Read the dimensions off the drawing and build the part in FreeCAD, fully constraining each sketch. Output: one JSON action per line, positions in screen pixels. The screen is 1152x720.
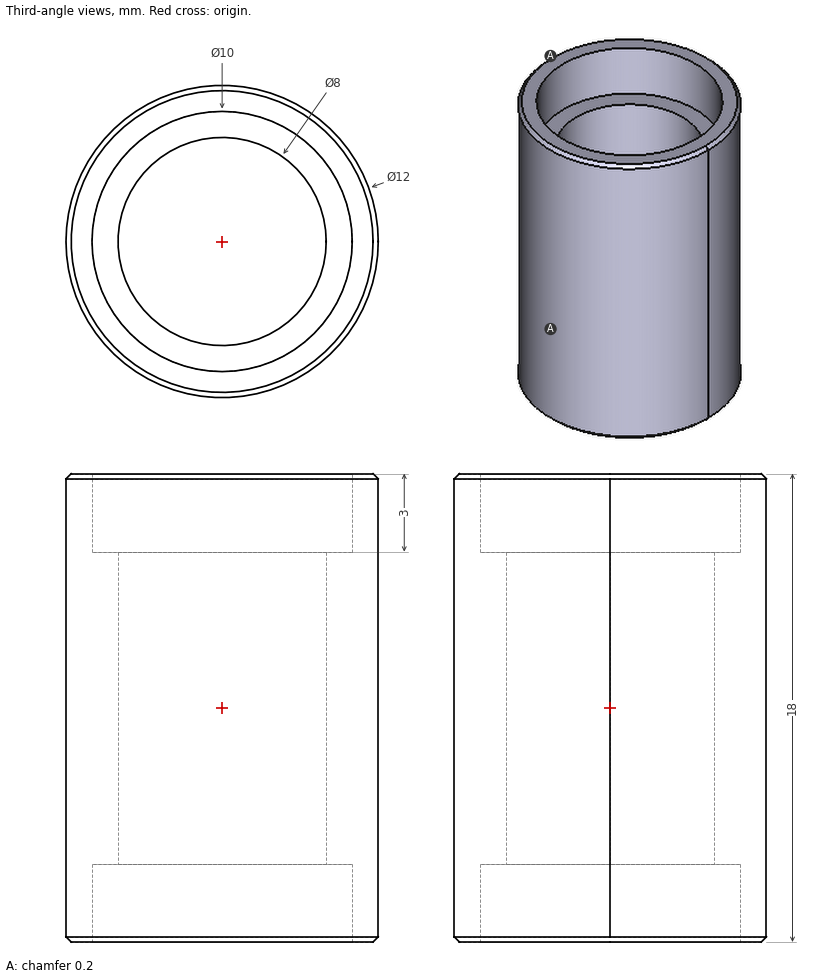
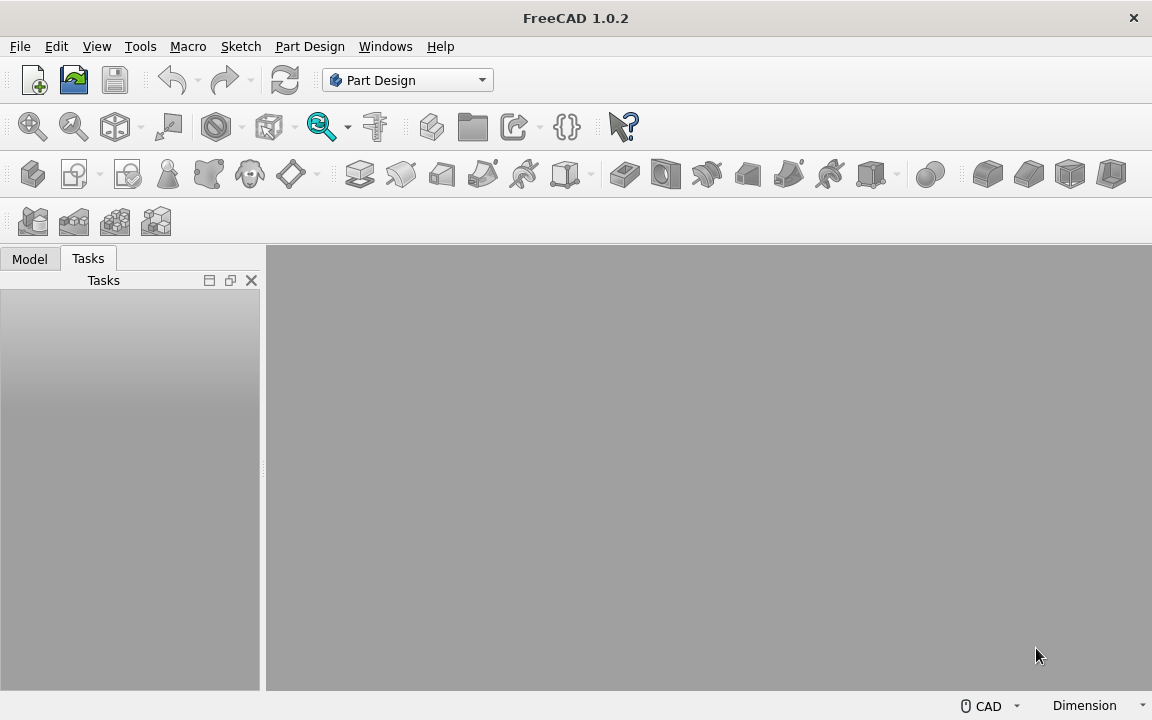
{"action": "left_click", "coordinate": [33, 80]}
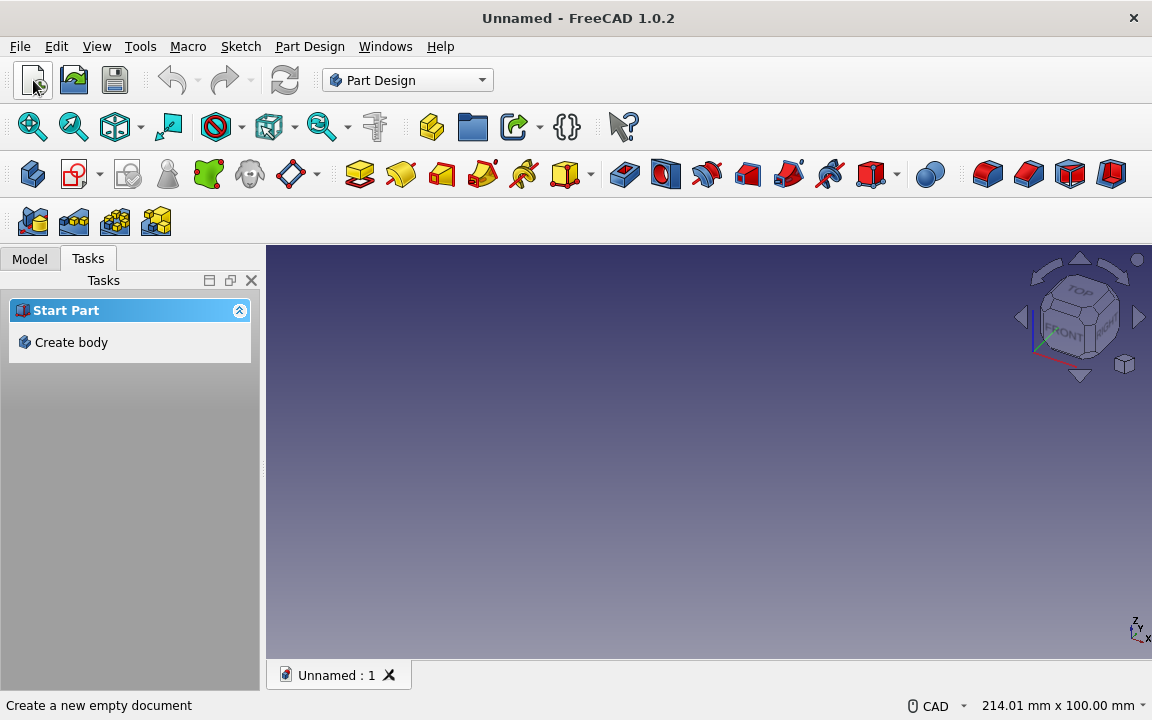
{"action": "left_click", "coordinate": [74, 174]}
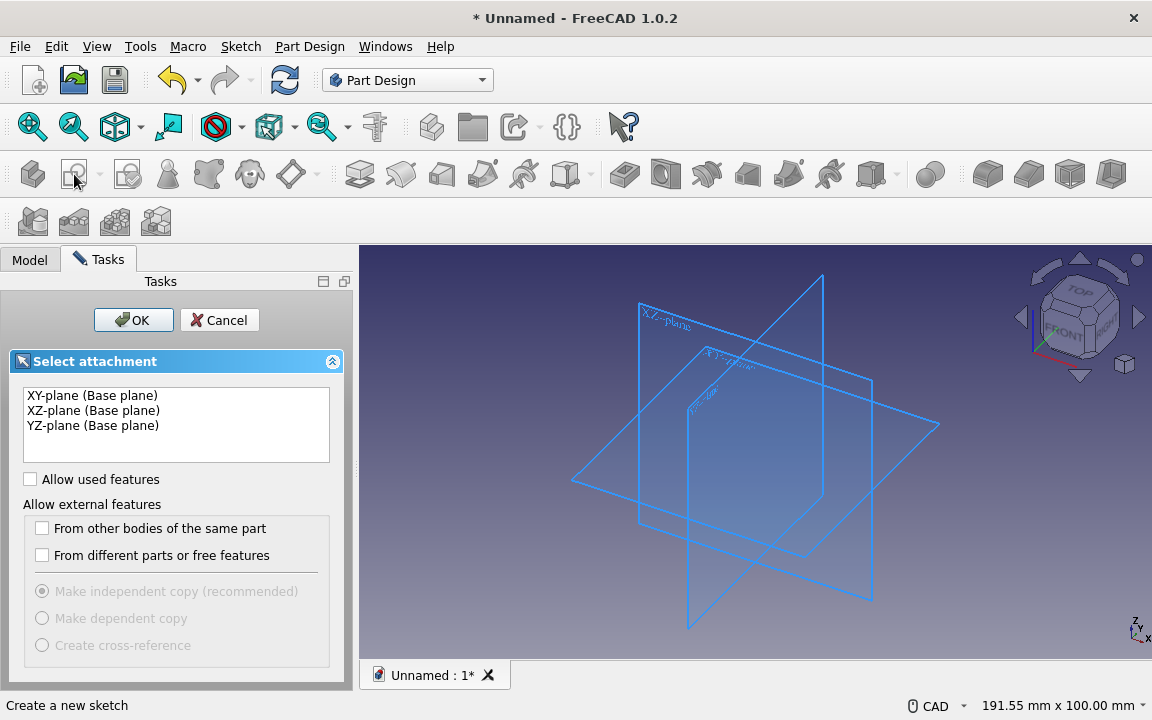
{"action": "left_click", "coordinate": [84, 396]}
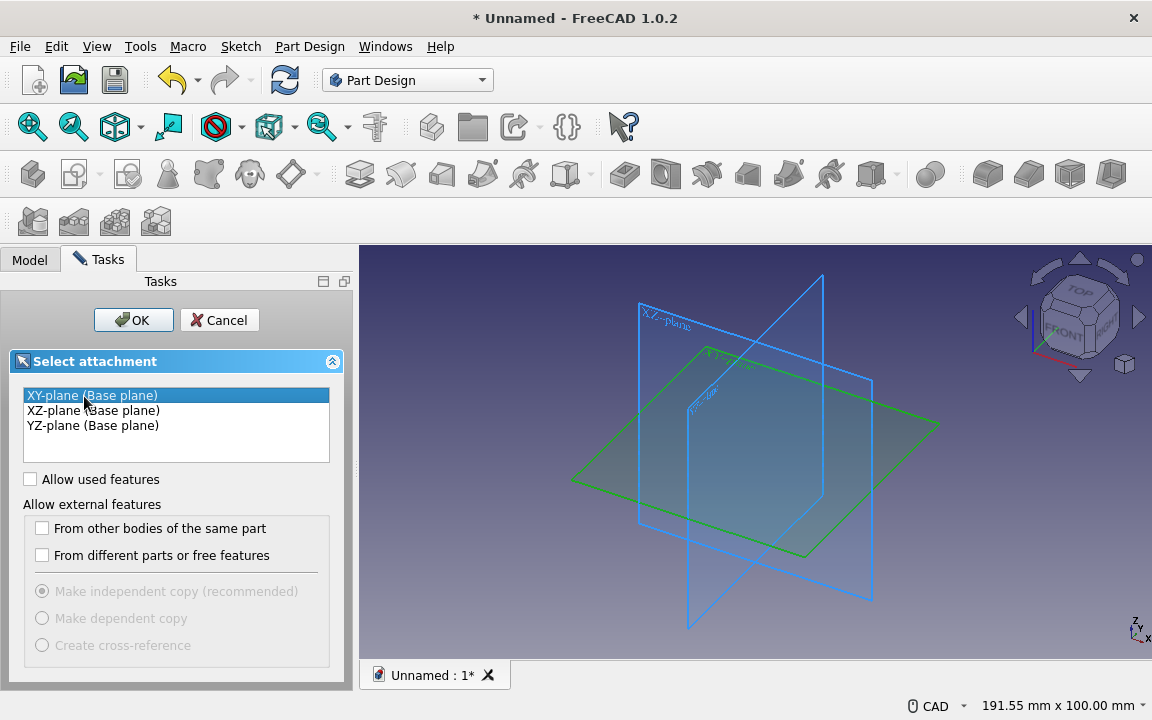
{"action": "left_click", "coordinate": [134, 320]}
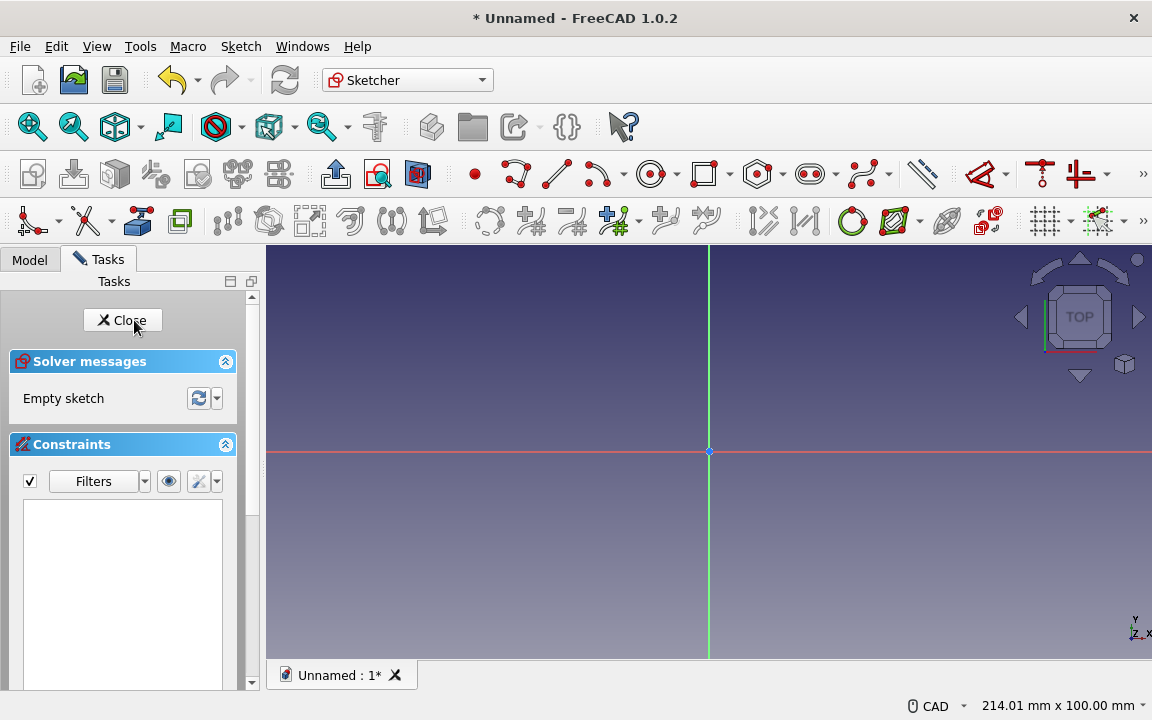
{"action": "scroll", "coordinate": [726, 452], "scroll_direction": "up", "scroll_amount": 8}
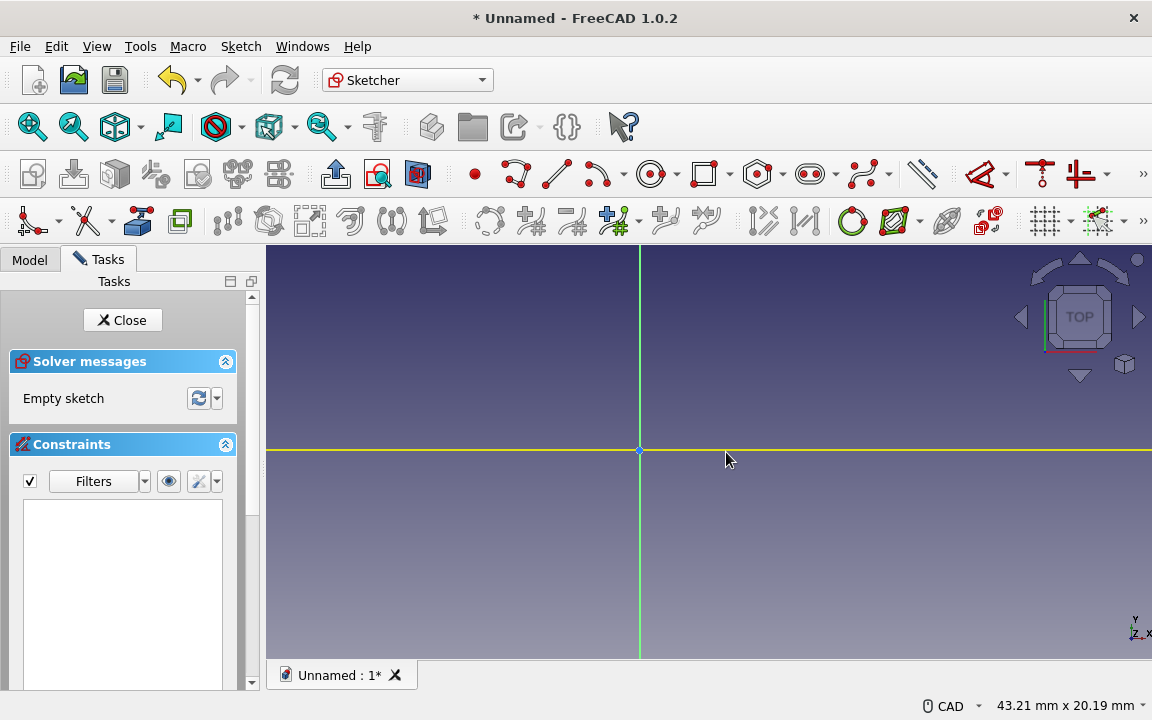
{"action": "left_click", "coordinate": [650, 174]}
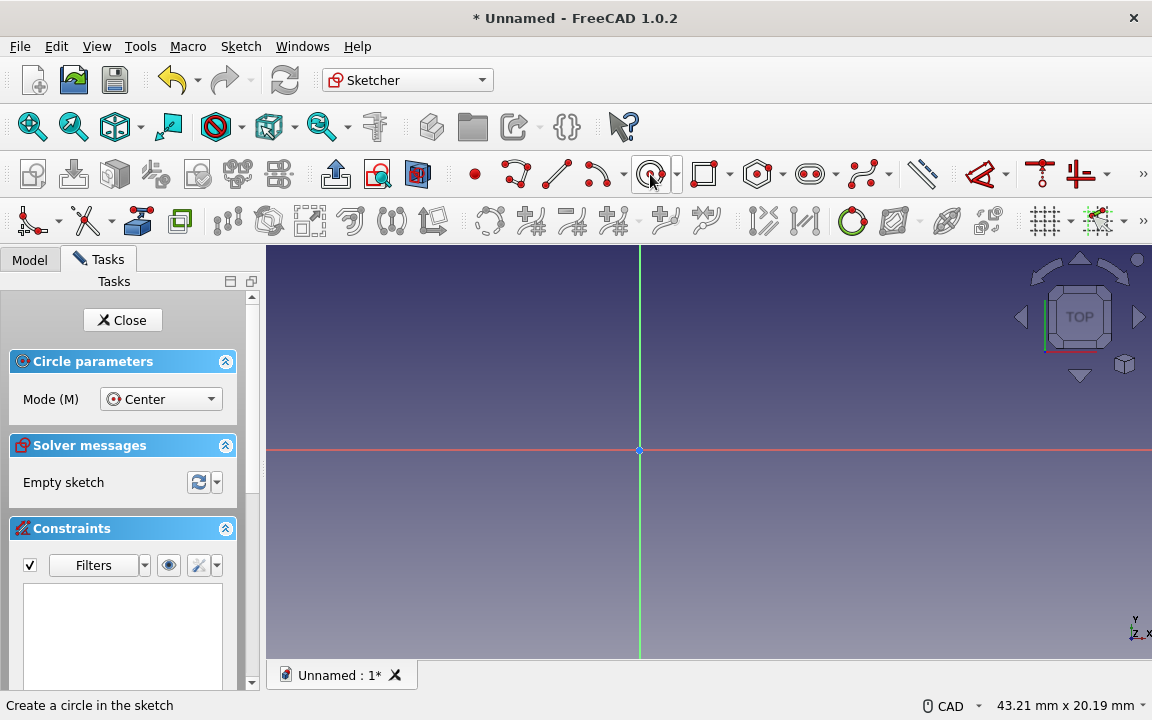
{"action": "left_click", "coordinate": [640, 450]}
{"action": "left_click", "coordinate": [727, 363]}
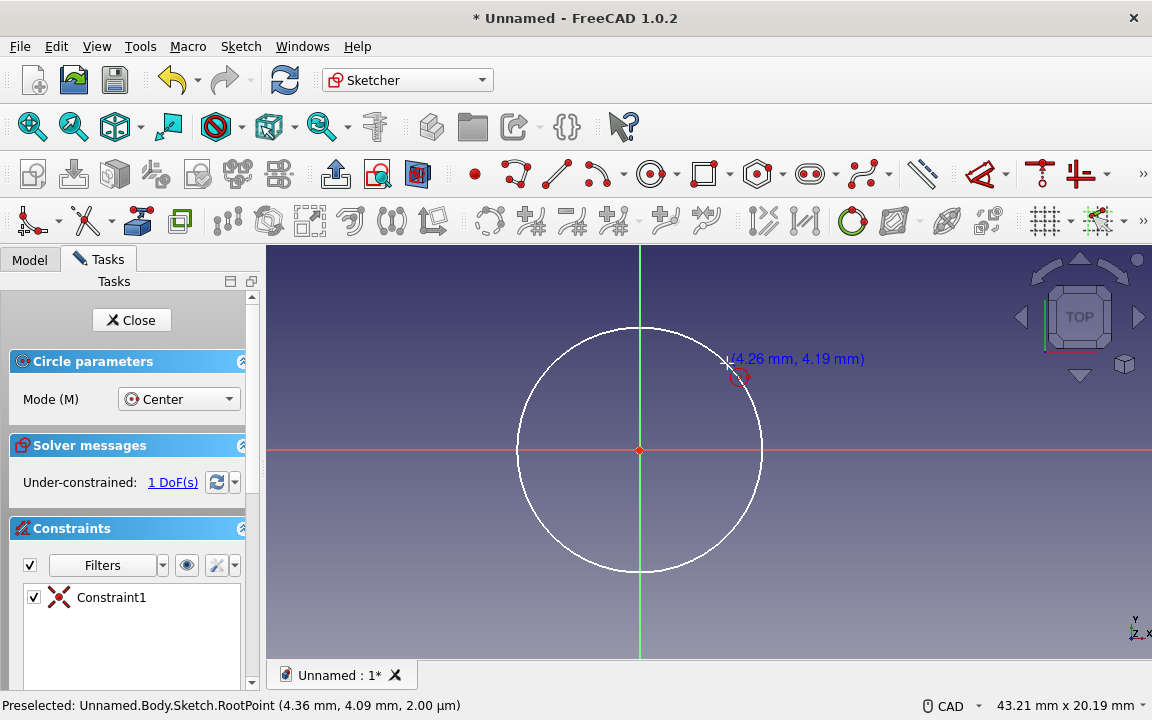
{"action": "left_click", "coordinate": [640, 450]}
{"action": "left_click", "coordinate": [698, 392]}
{"action": "key", "text": "Escape"}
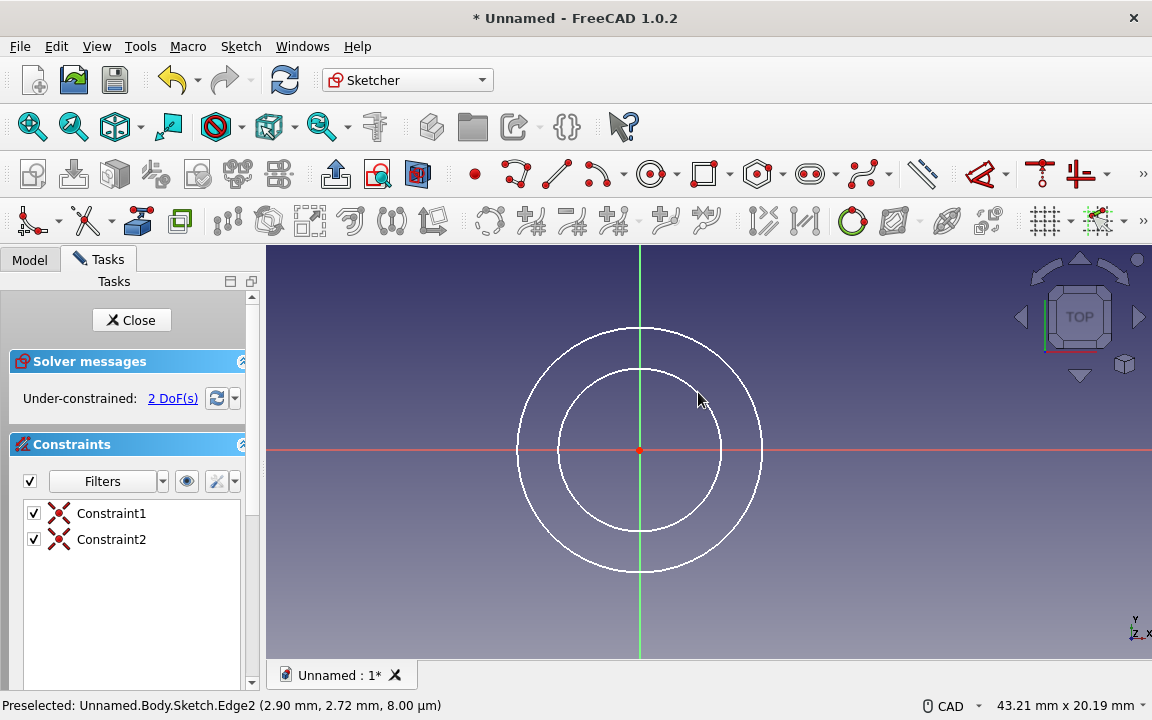
{"action": "key", "text": "d"}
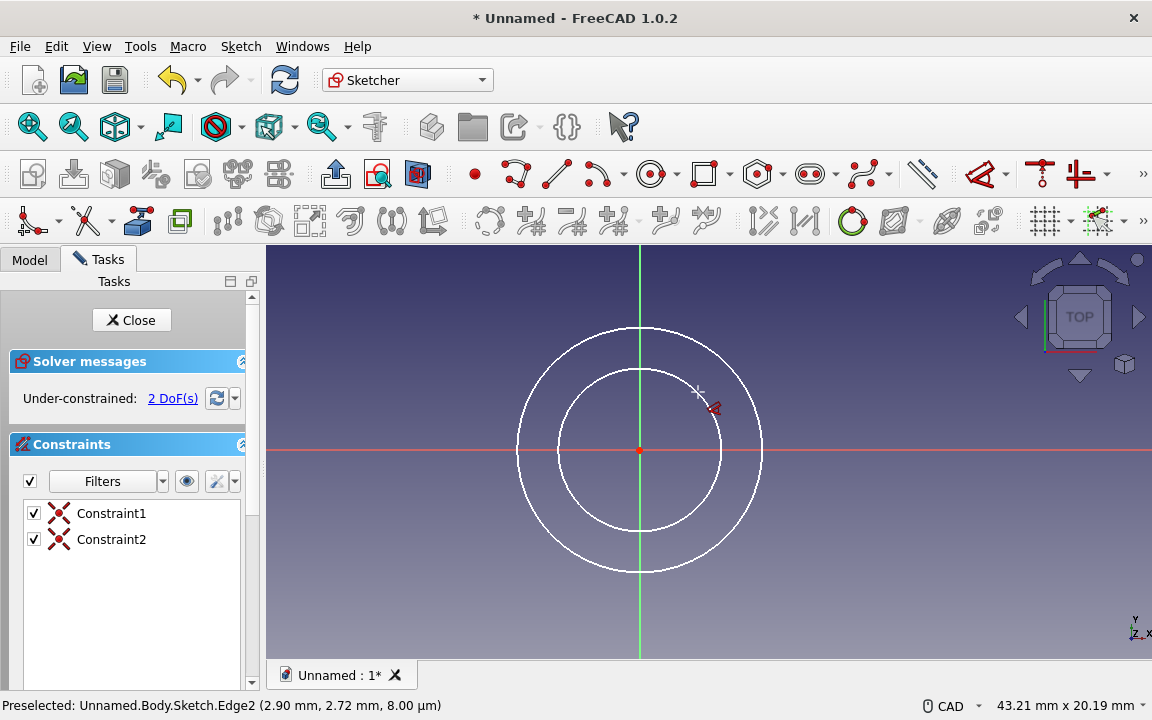
{"action": "left_click", "coordinate": [726, 363]}
{"action": "left_click", "coordinate": [749, 340]}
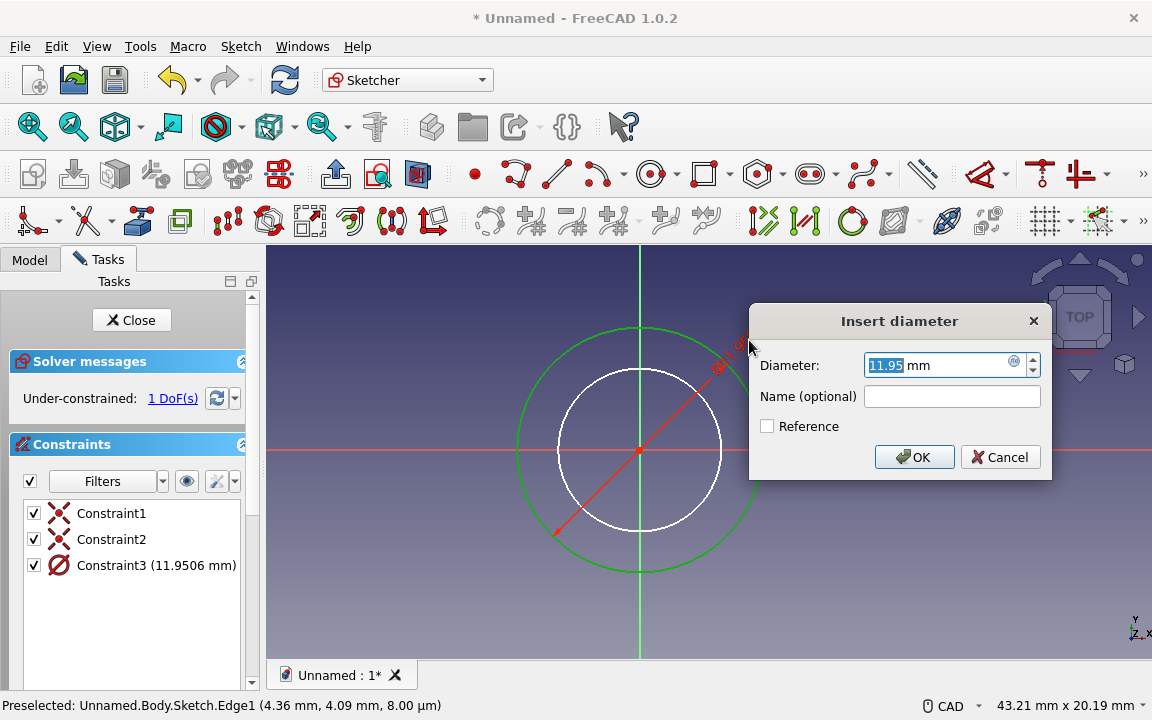
{"action": "type", "text": "12"}
{"action": "key", "text": "Return"}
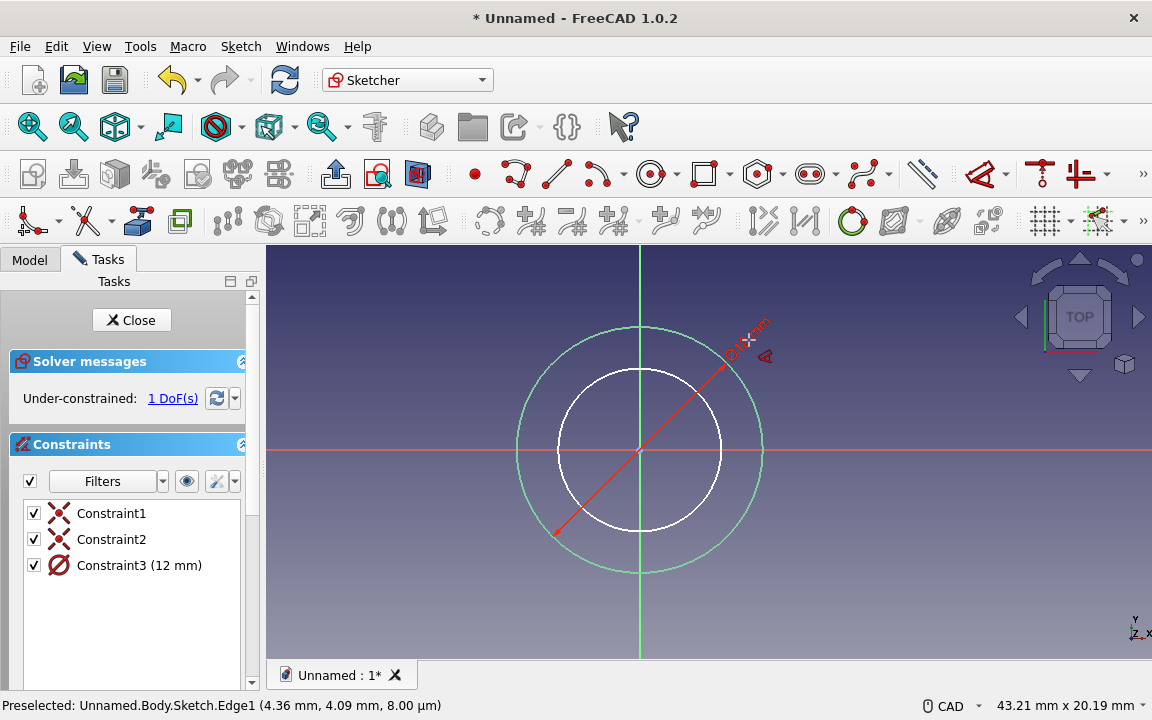
{"action": "left_click", "coordinate": [697, 392]}
{"action": "left_click", "coordinate": [770, 411]}